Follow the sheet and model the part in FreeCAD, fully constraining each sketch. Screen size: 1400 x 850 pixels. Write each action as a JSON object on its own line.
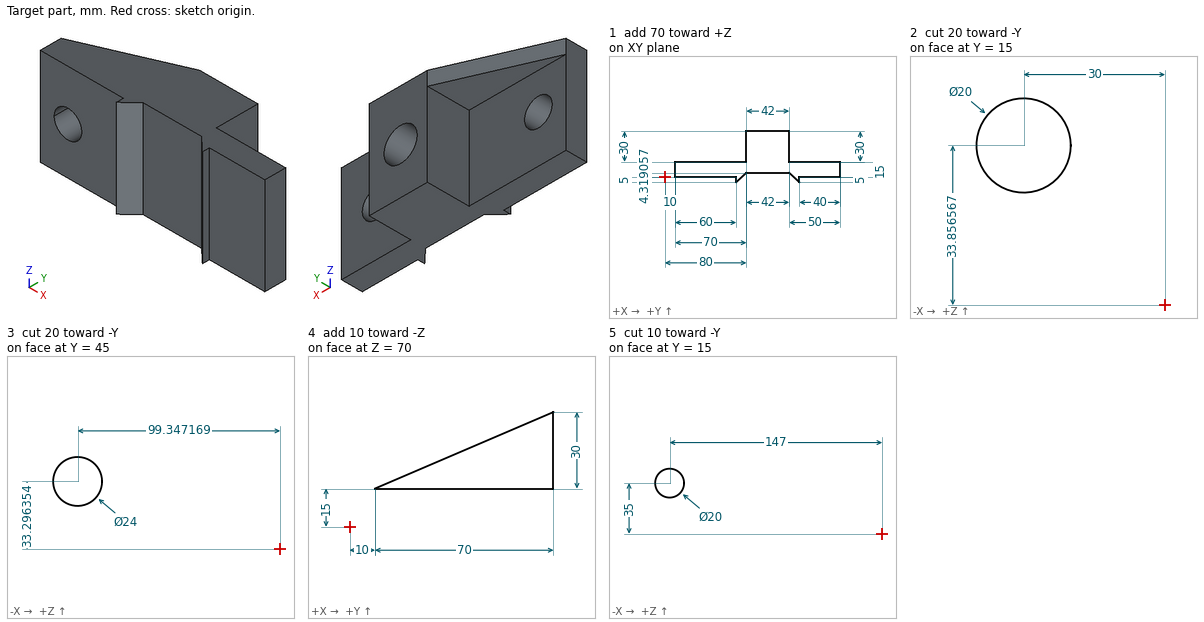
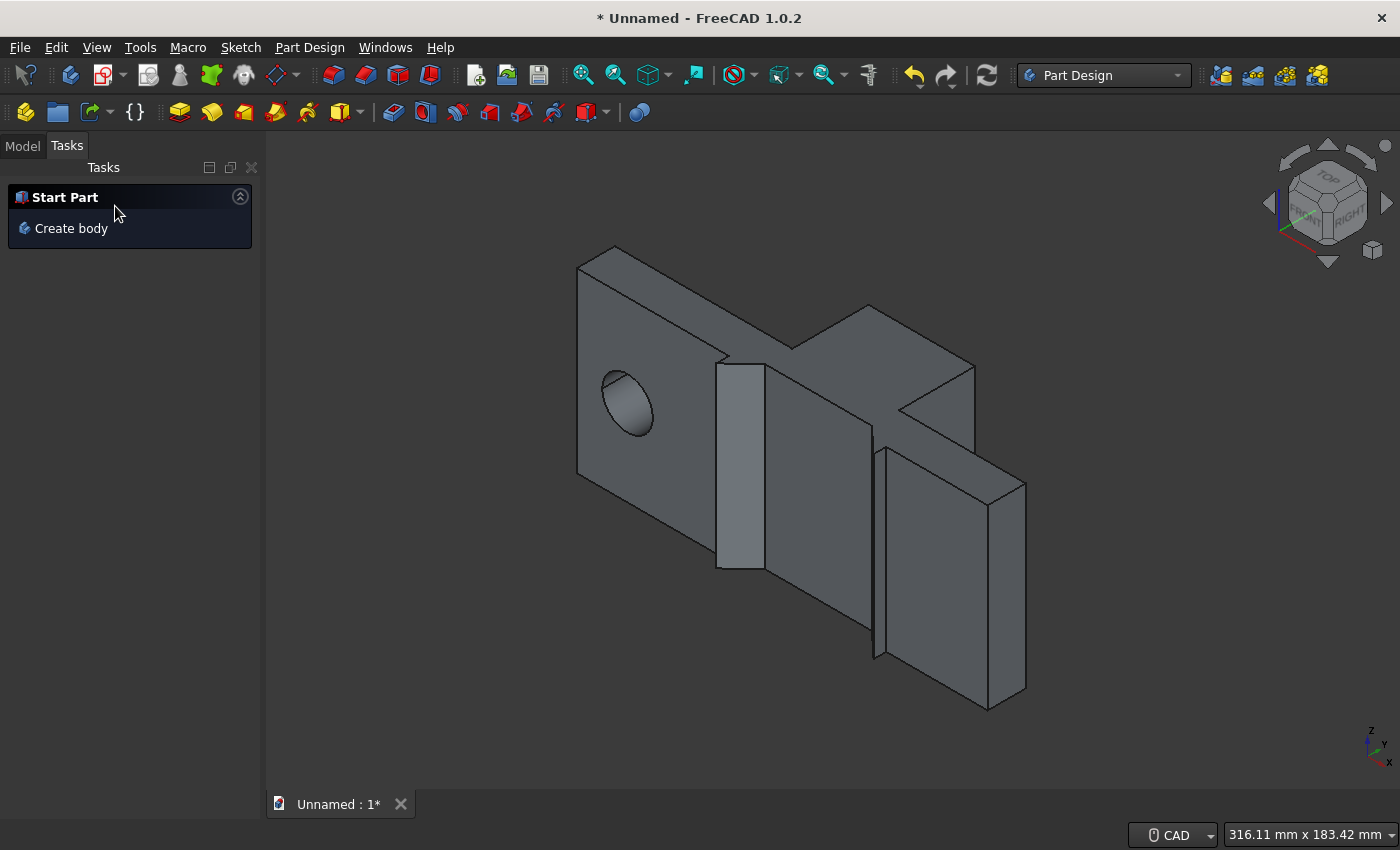
{"action": "left_click", "coordinate": [851, 346]}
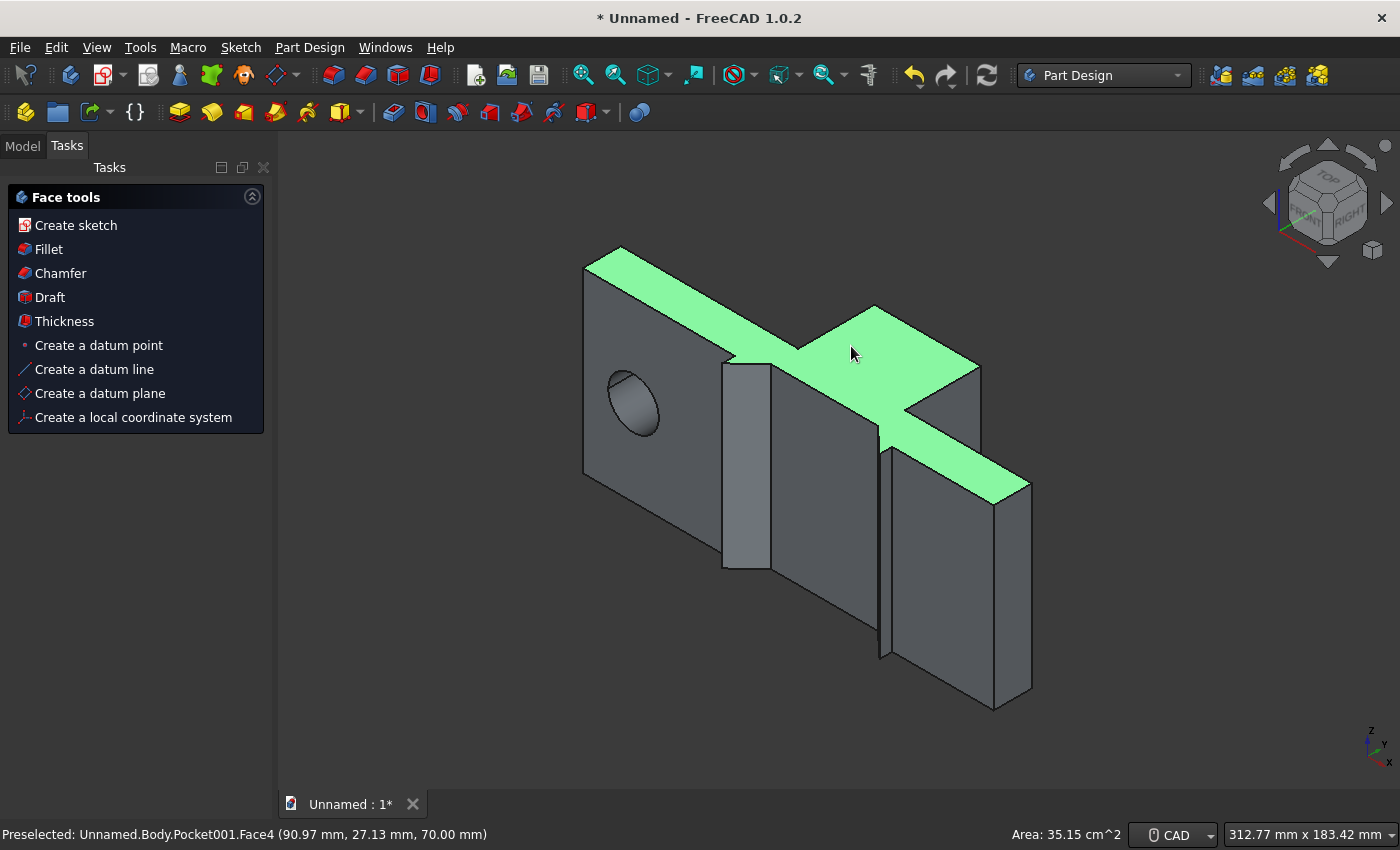
{"action": "left_click", "coordinate": [104, 76]}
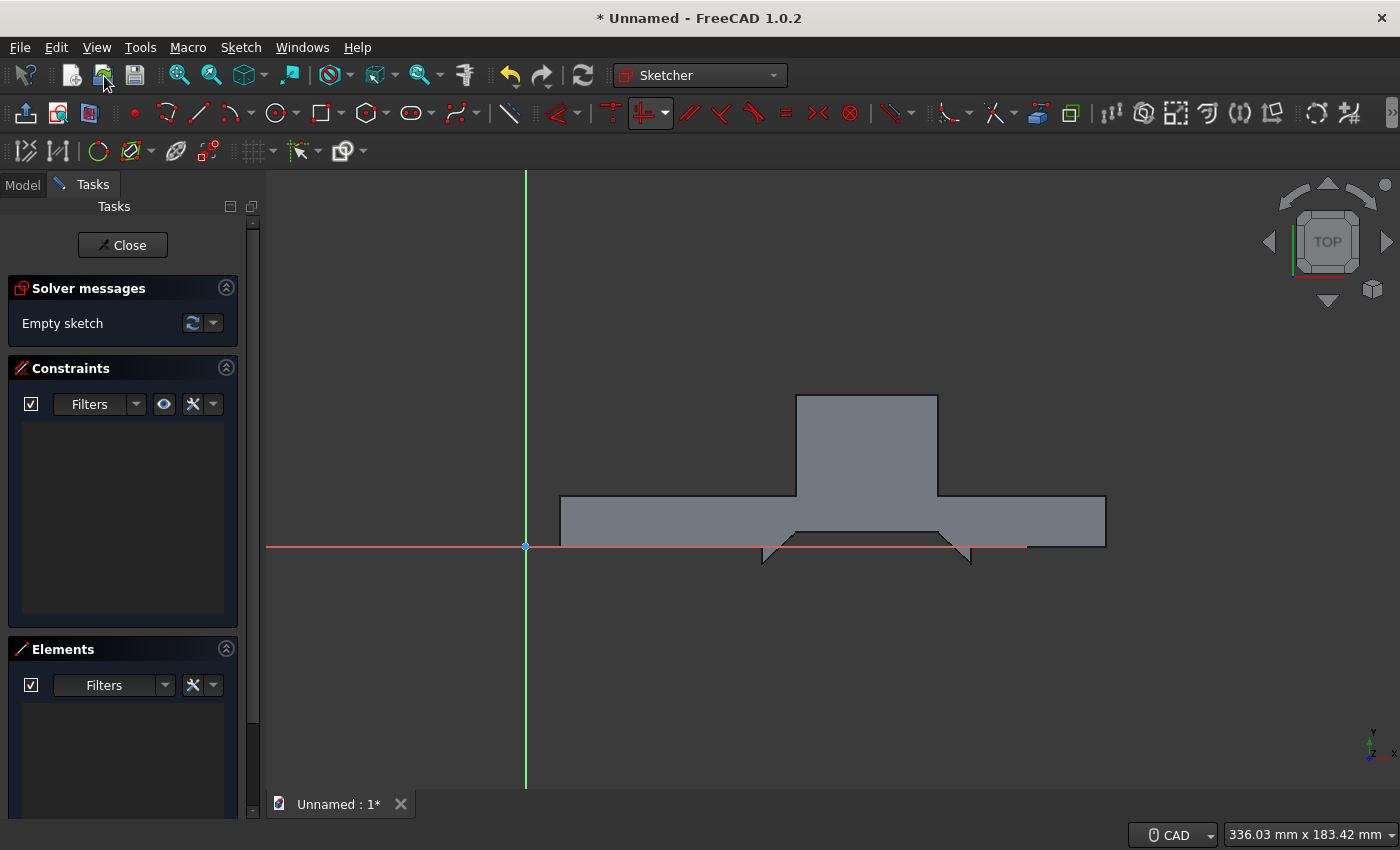
{"action": "scroll", "coordinate": [601, 466], "scroll_direction": "up", "scroll_amount": 5}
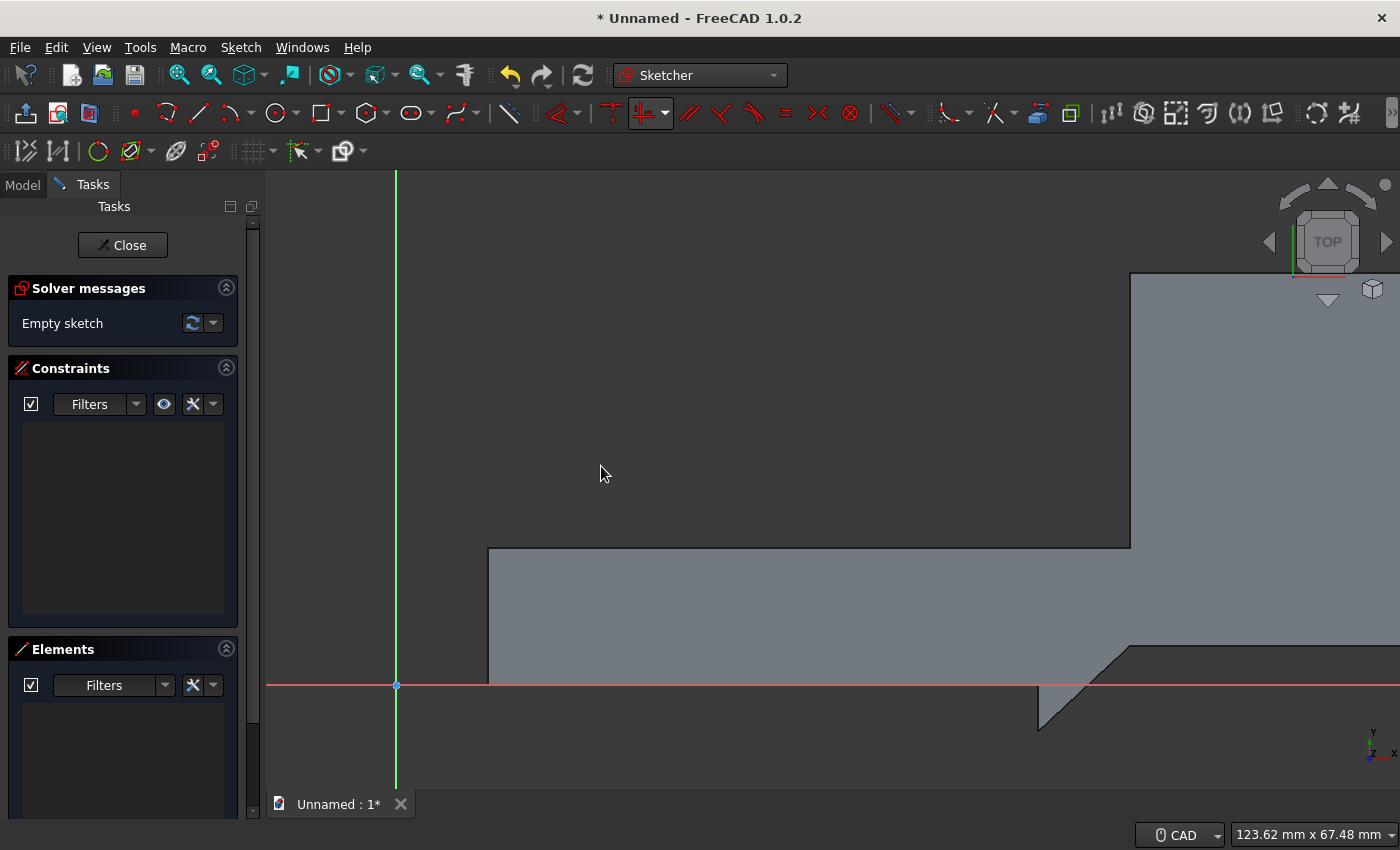
{"action": "left_click", "coordinate": [168, 114]}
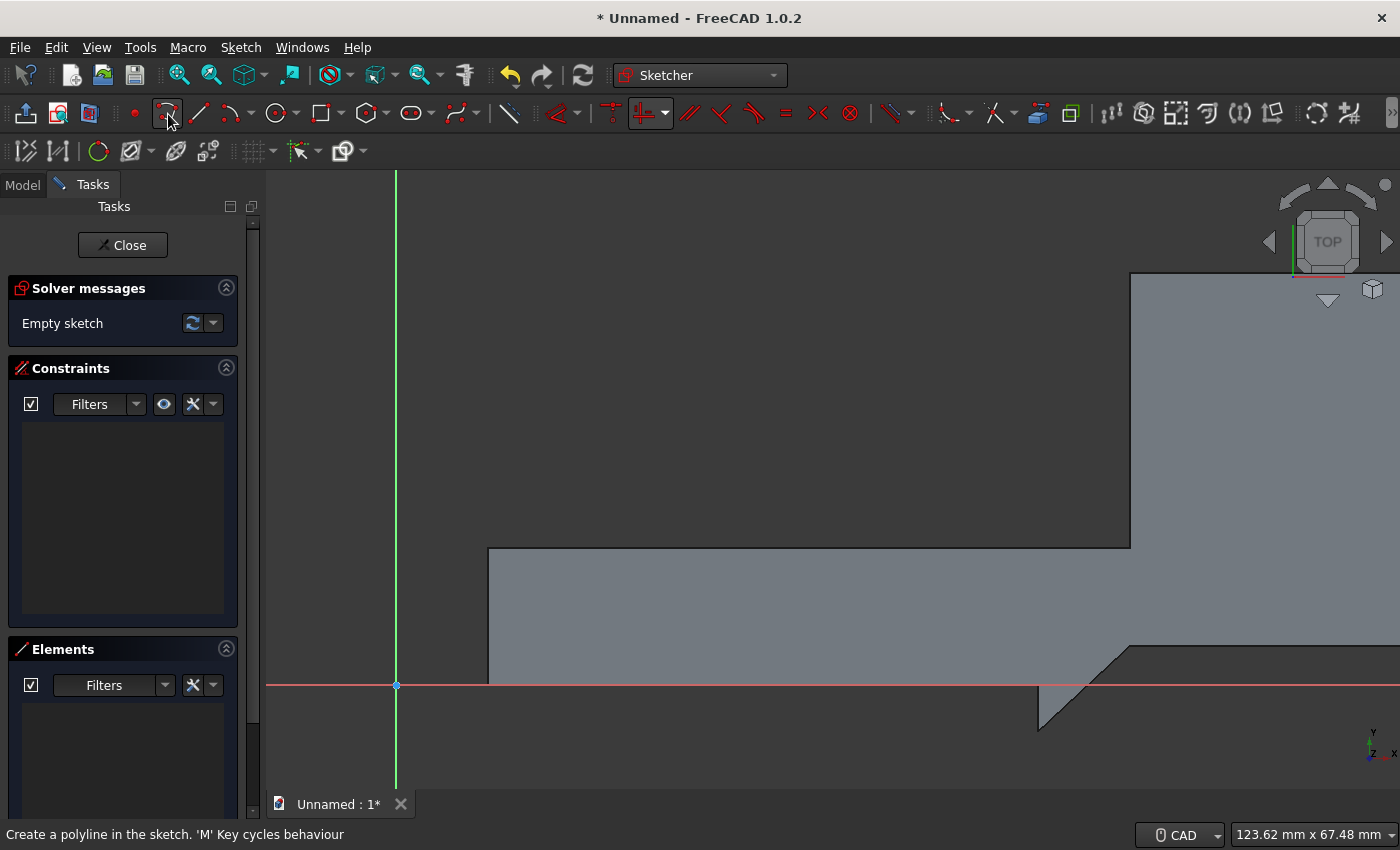
{"action": "left_click", "coordinate": [488, 548]}
{"action": "left_click", "coordinate": [1130, 548]}
{"action": "left_click", "coordinate": [1130, 273]}
{"action": "left_click", "coordinate": [488, 549]}
{"action": "key", "text": "Escape"}
{"action": "key", "text": "Escape"}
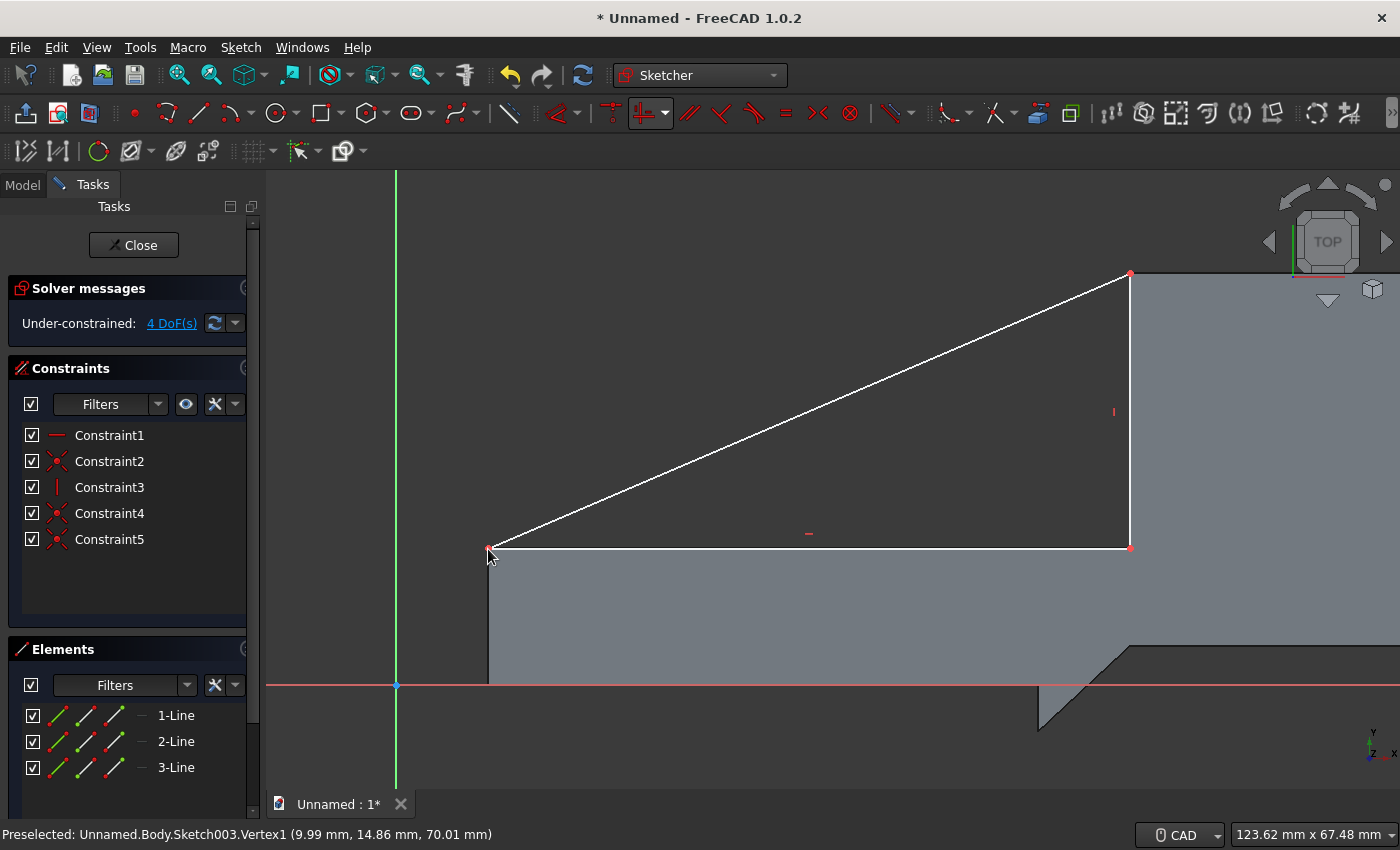
{"action": "left_click", "coordinate": [556, 114]}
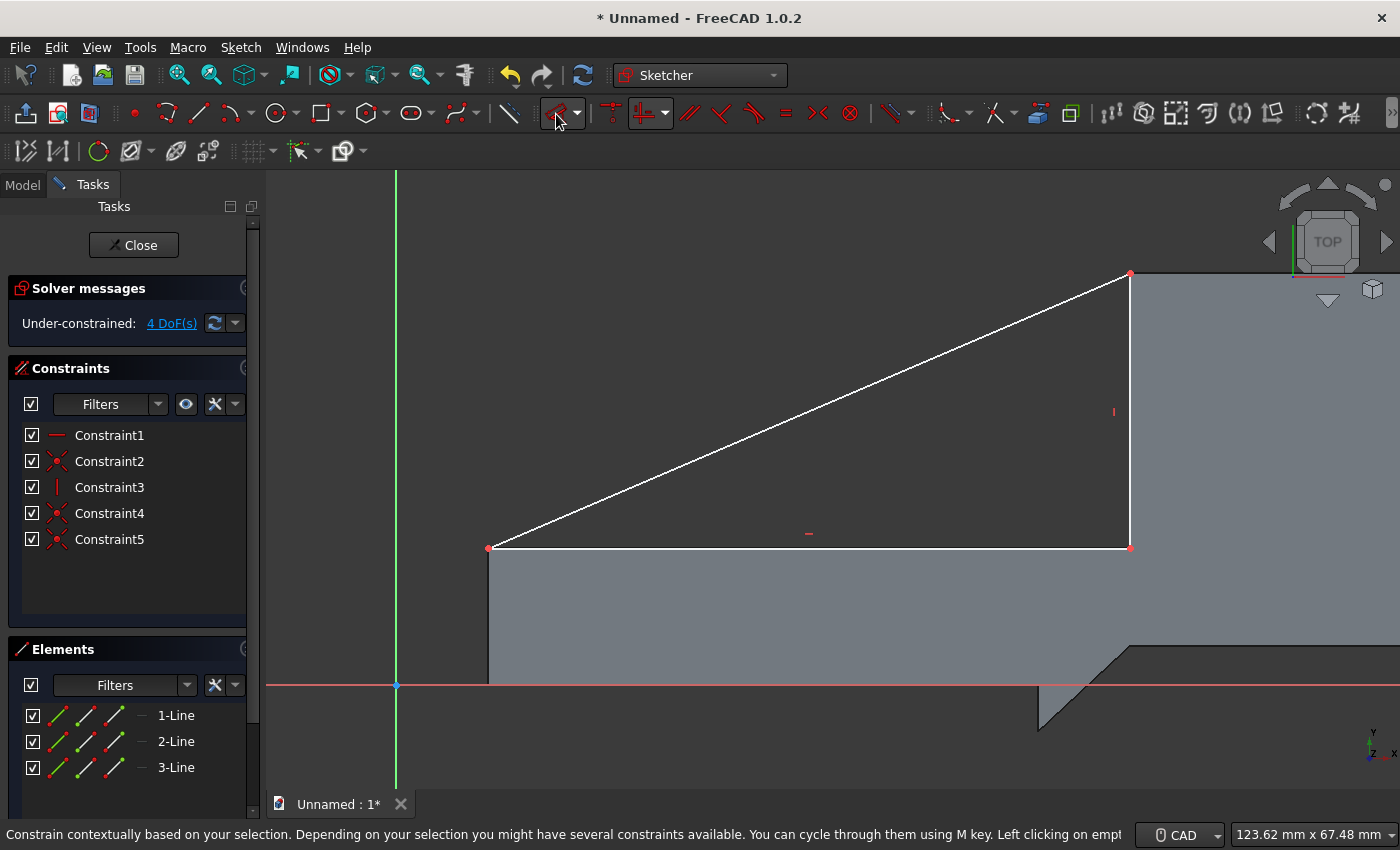
{"action": "left_click", "coordinate": [681, 549]}
{"action": "left_click", "coordinate": [809, 583]}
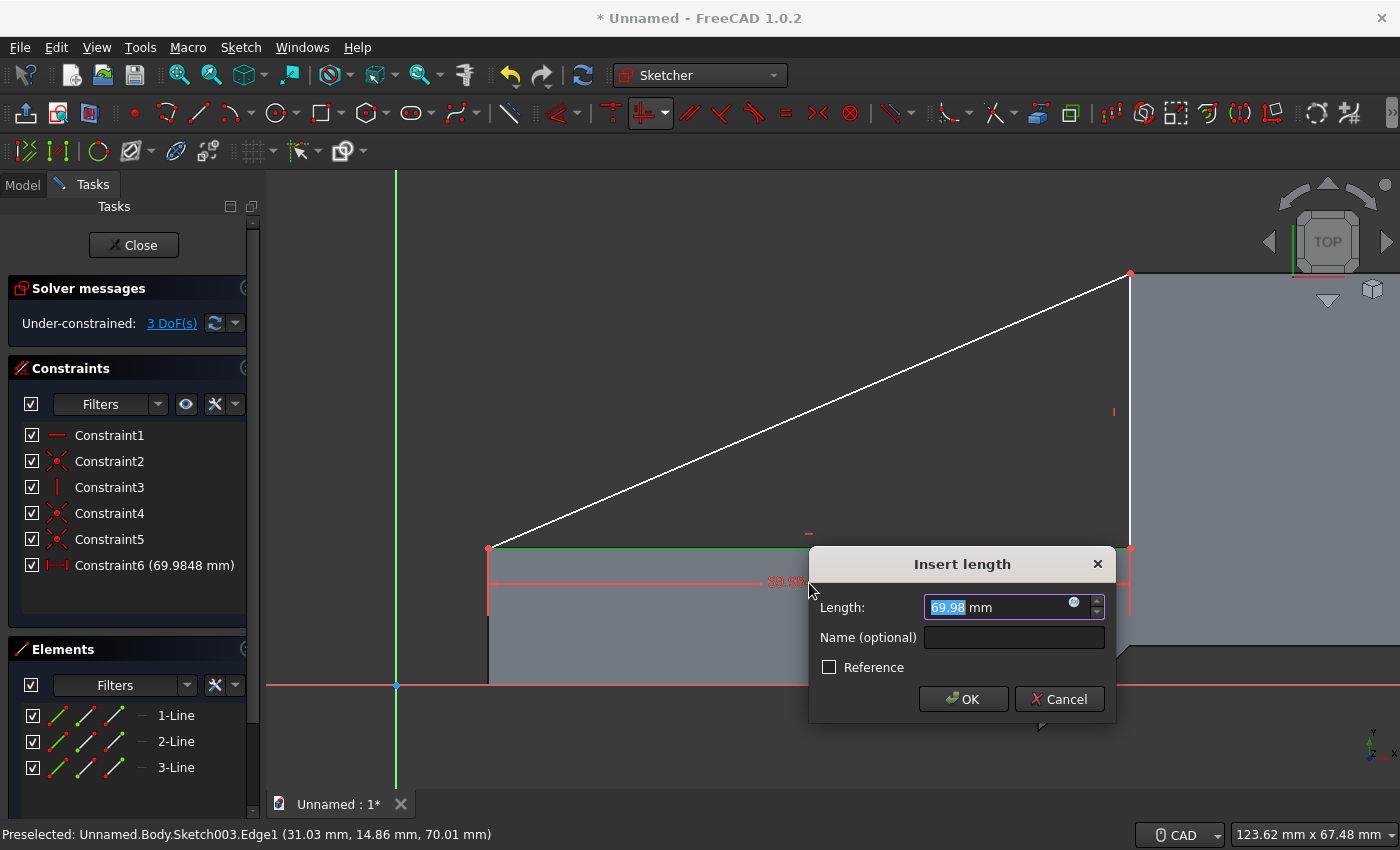
{"action": "type", "text": "70"}
{"action": "key", "text": "Return"}